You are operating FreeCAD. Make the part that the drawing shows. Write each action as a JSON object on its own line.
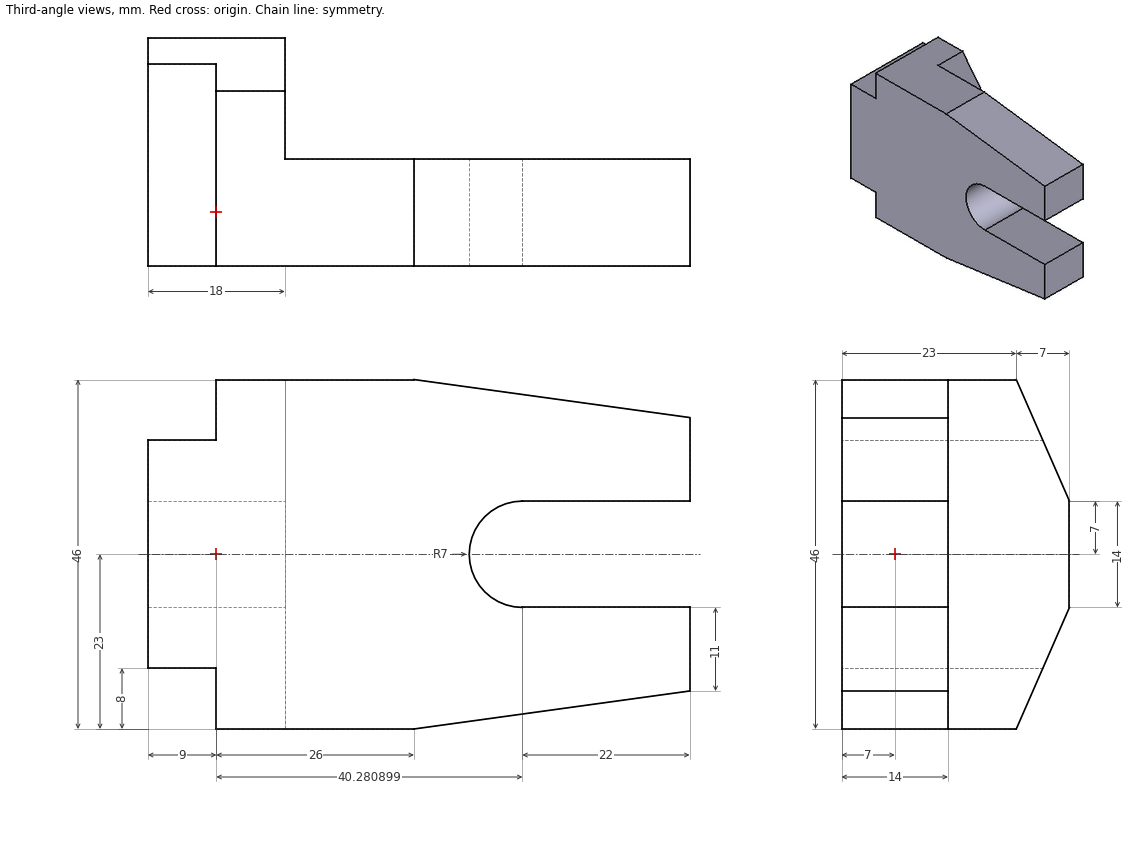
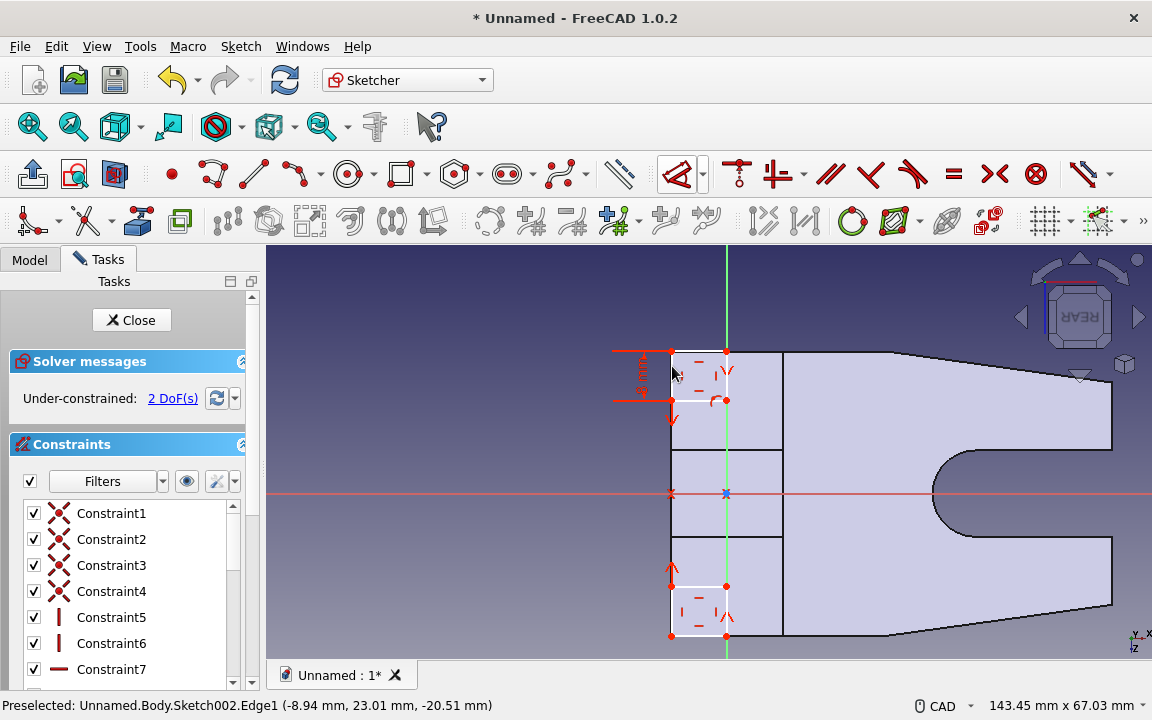
{"action": "left_click", "coordinate": [688, 401]}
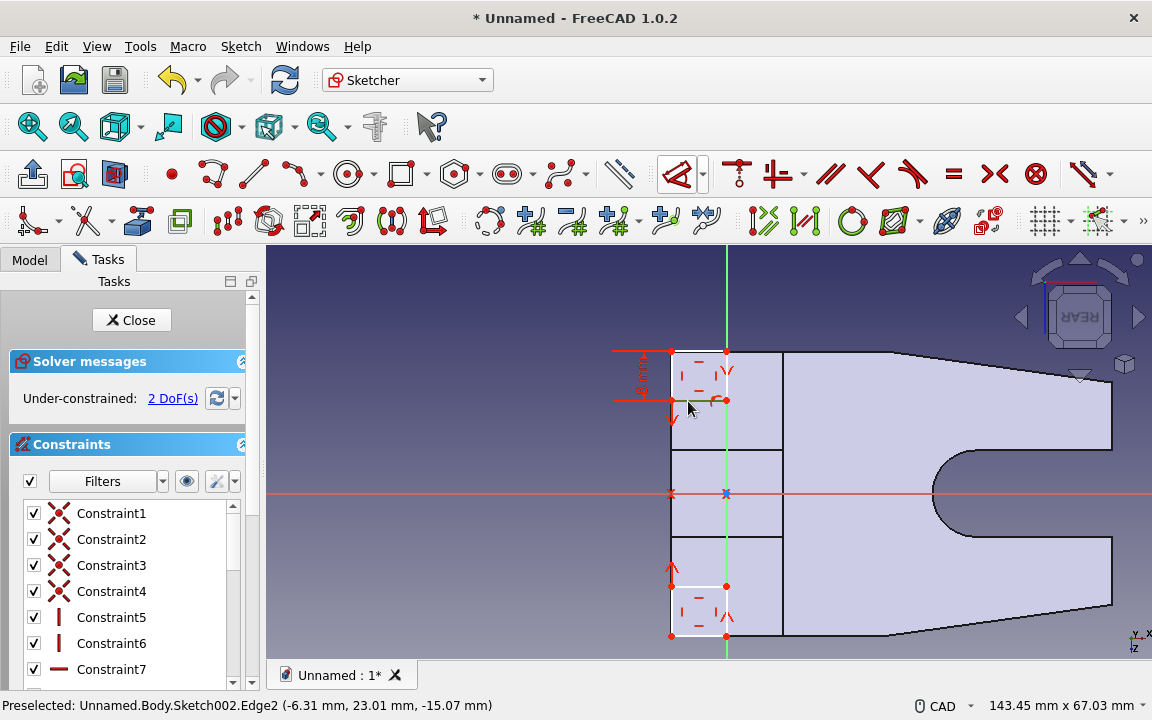
{"action": "key", "text": "l"}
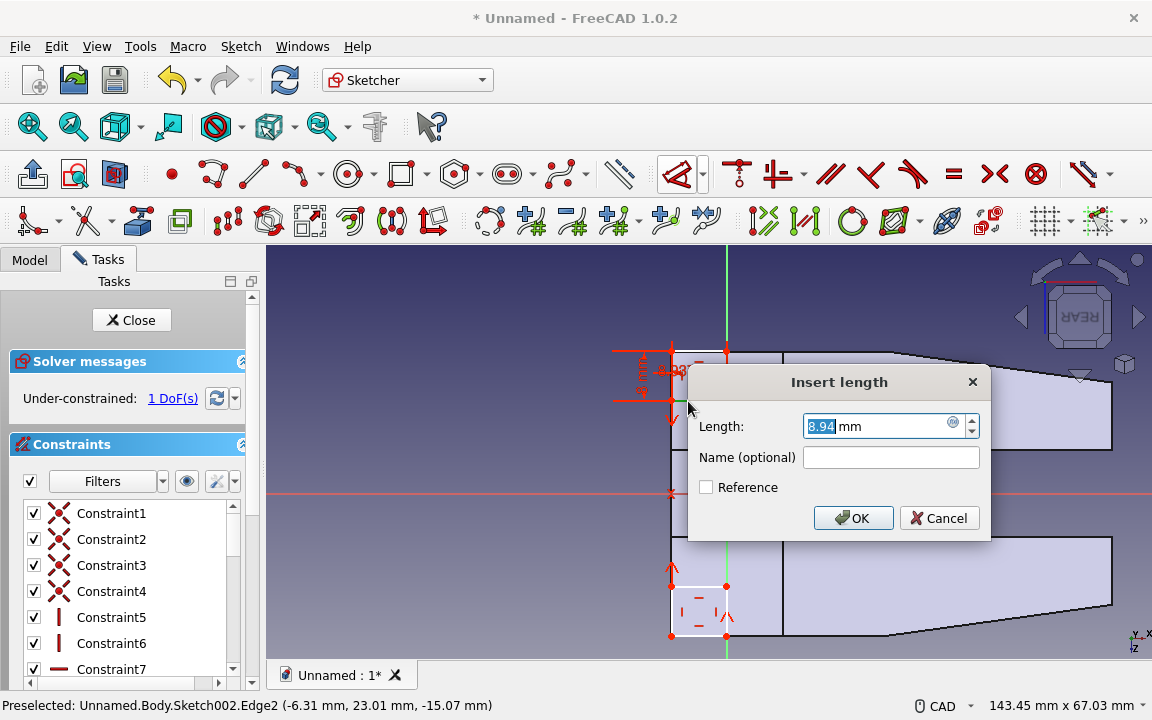
{"action": "type", "text": "9"}
{"action": "key", "text": "Return"}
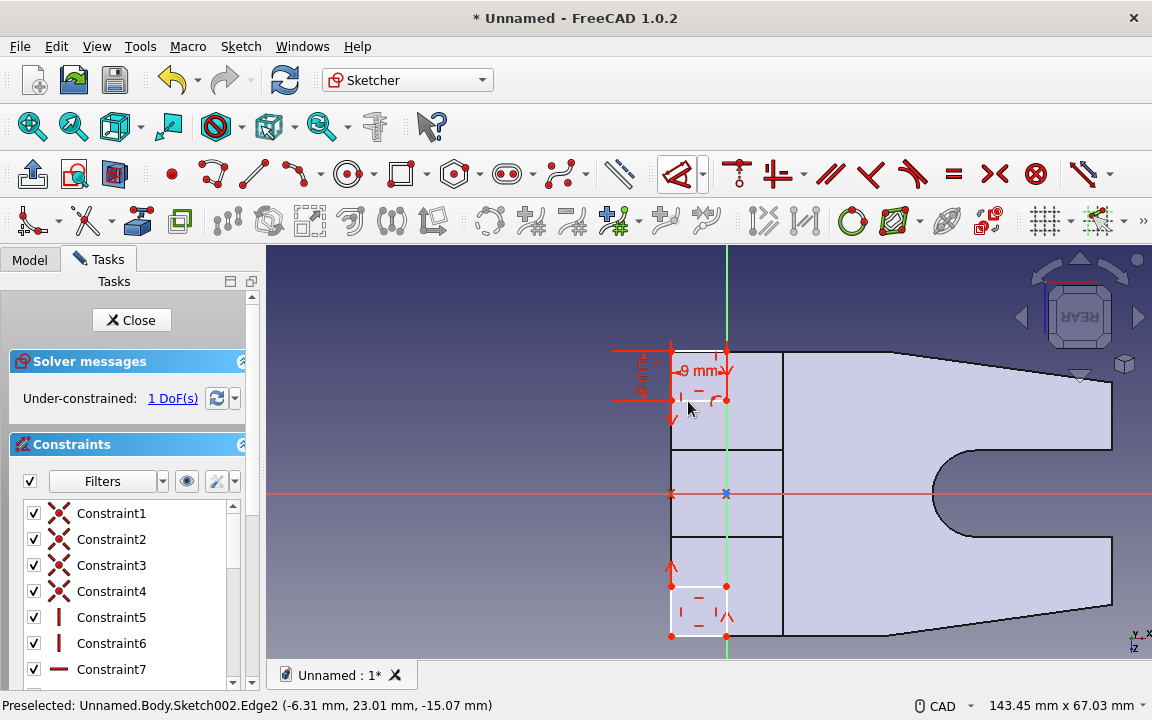
{"action": "left_click", "coordinate": [671, 351]}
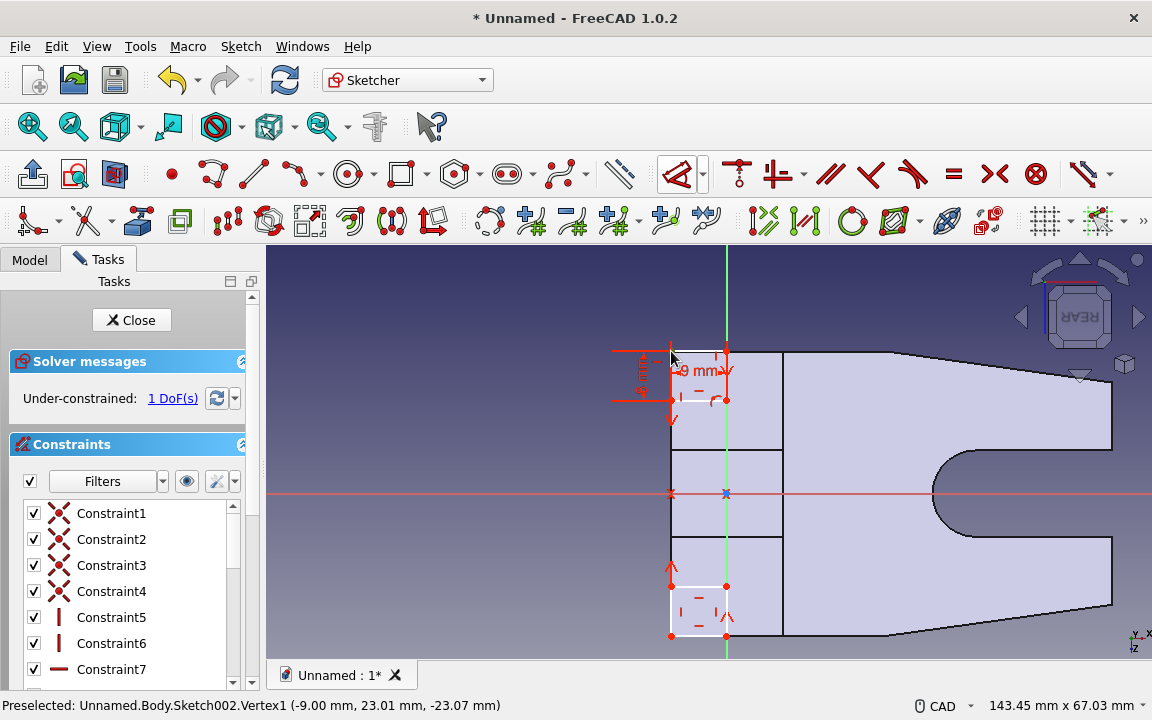
{"action": "key", "text": "i"}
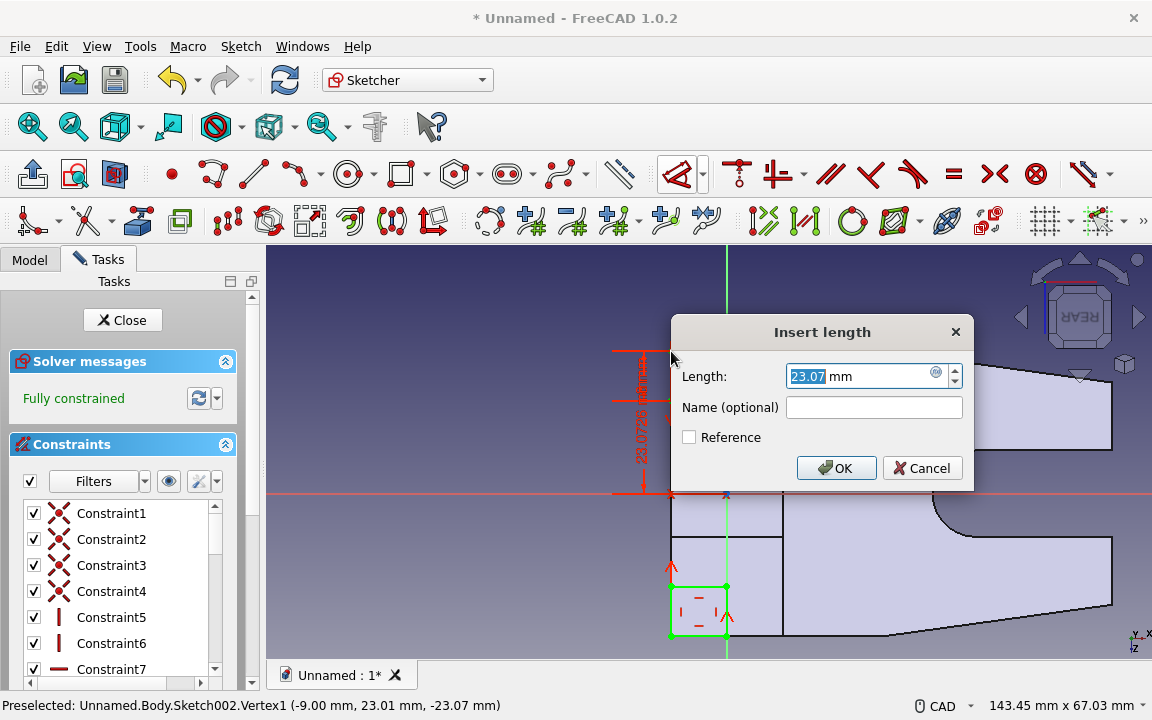
{"action": "type", "text": "23"}
{"action": "key", "text": "Return"}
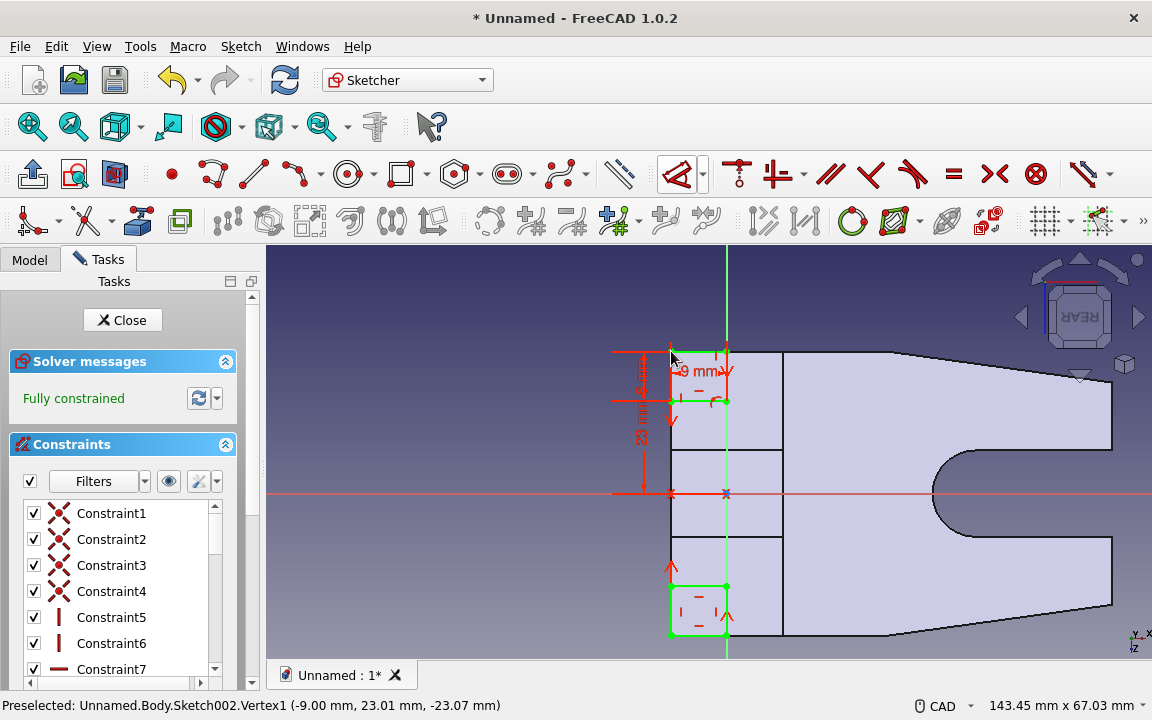
{"action": "left_click", "coordinate": [123, 320]}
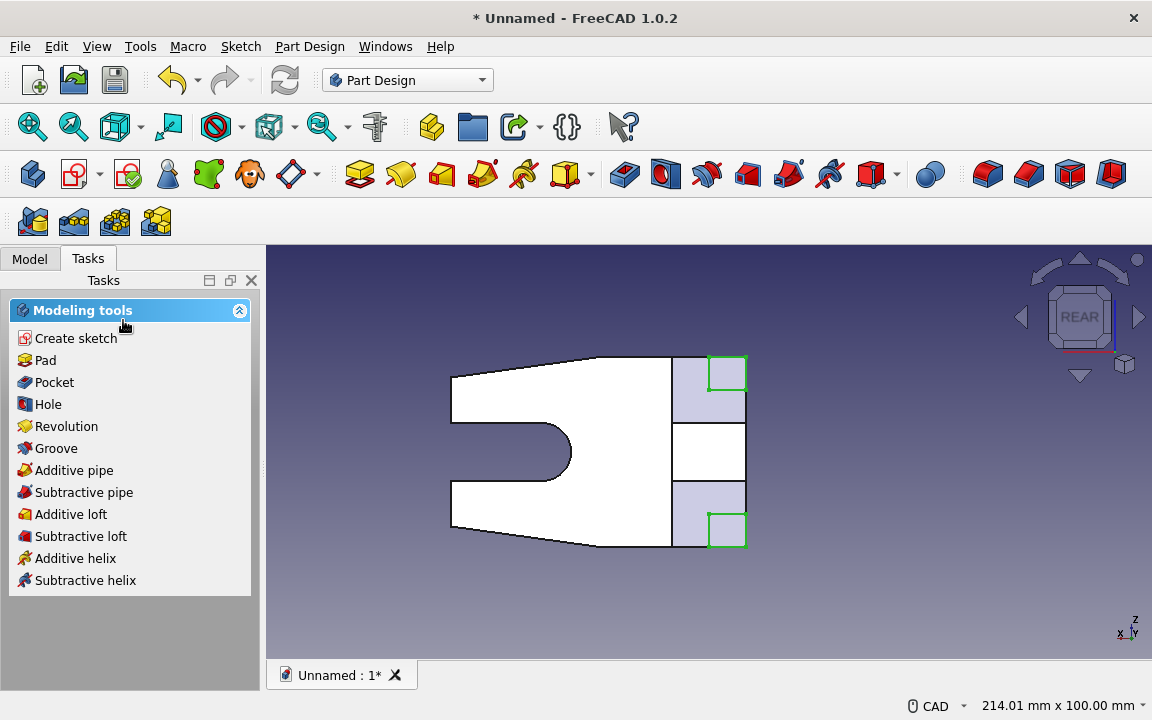
{"action": "left_click", "coordinate": [625, 174]}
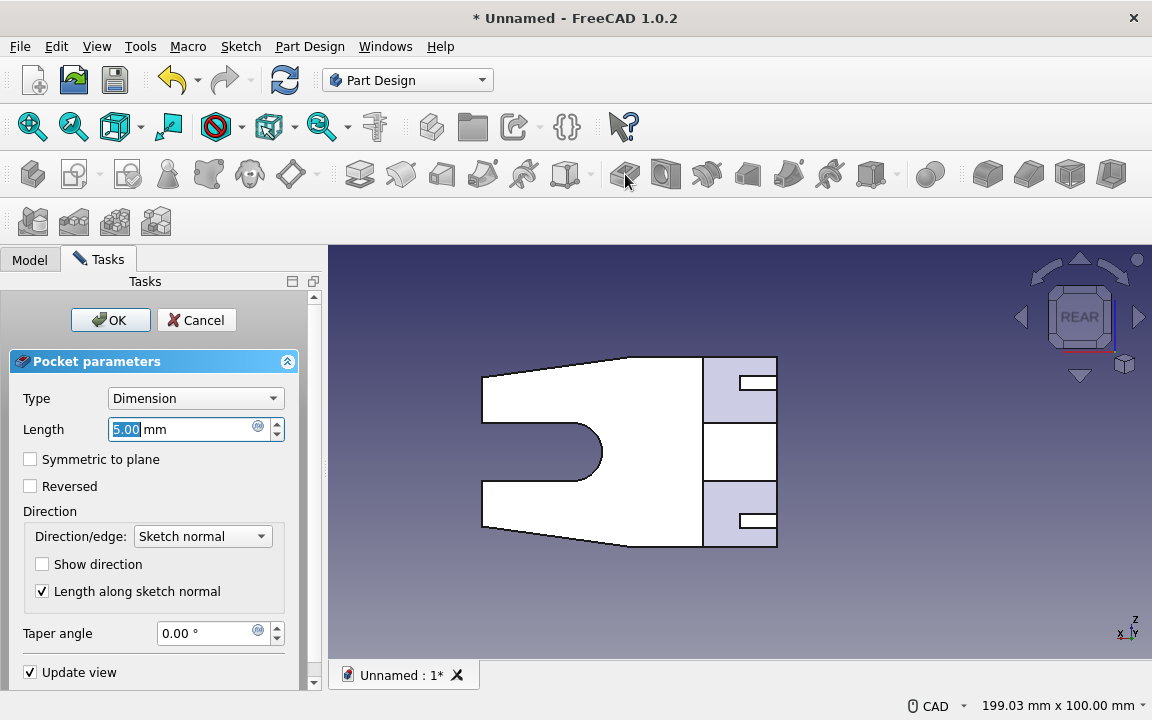
{"action": "left_click", "coordinate": [196, 398]}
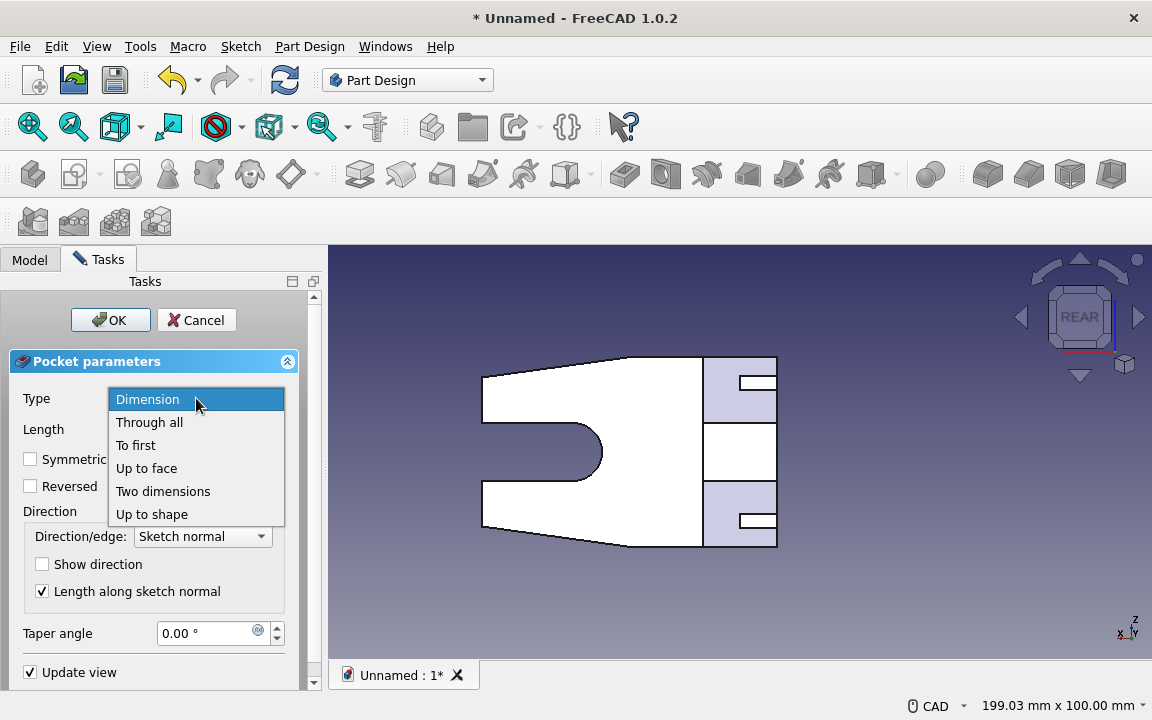
{"action": "left_click", "coordinate": [194, 422]}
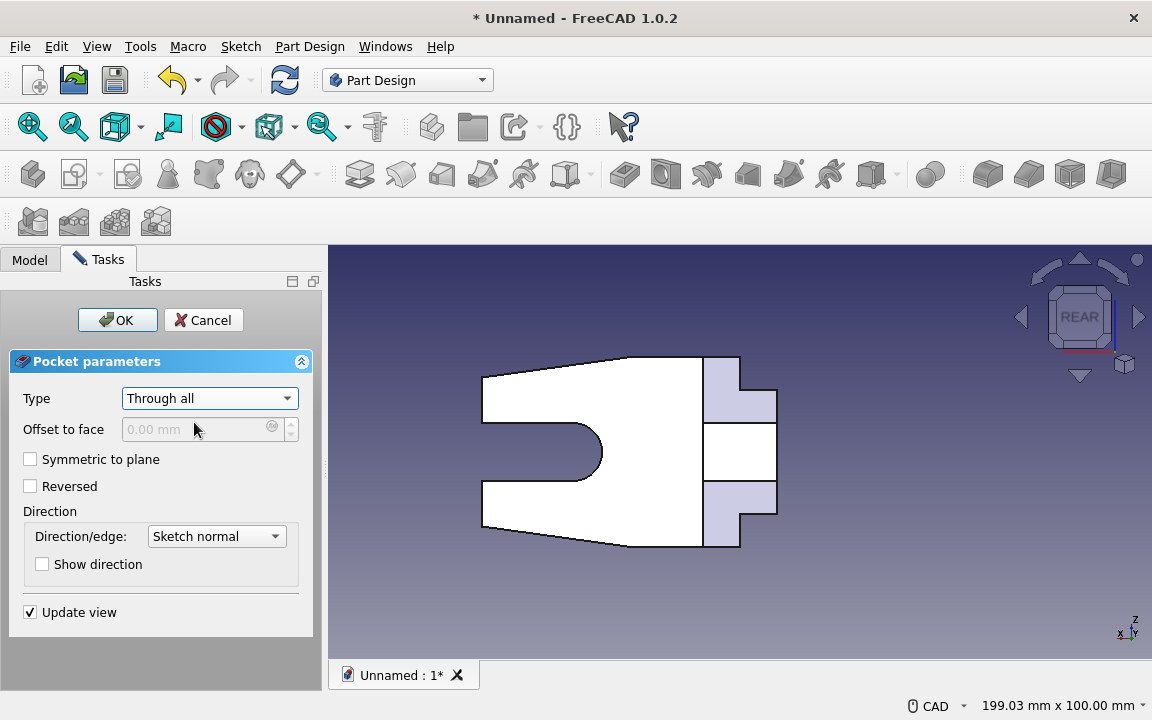
{"action": "left_click", "coordinate": [118, 320]}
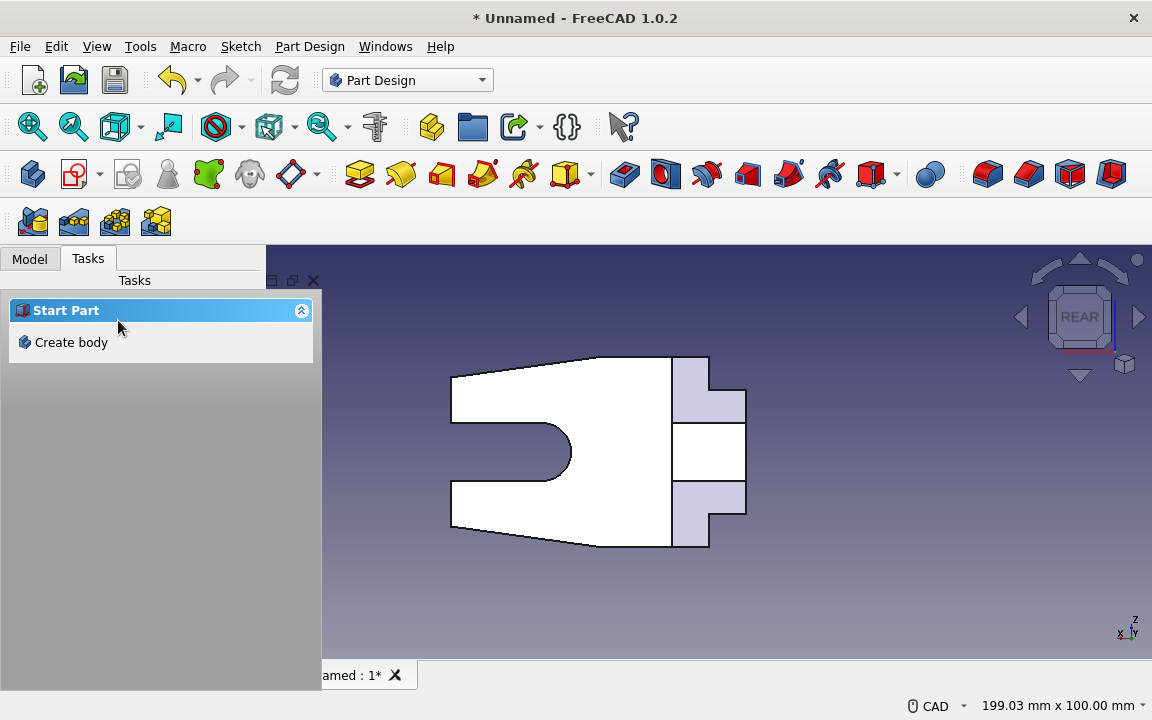
{"action": "key", "text": "0"}